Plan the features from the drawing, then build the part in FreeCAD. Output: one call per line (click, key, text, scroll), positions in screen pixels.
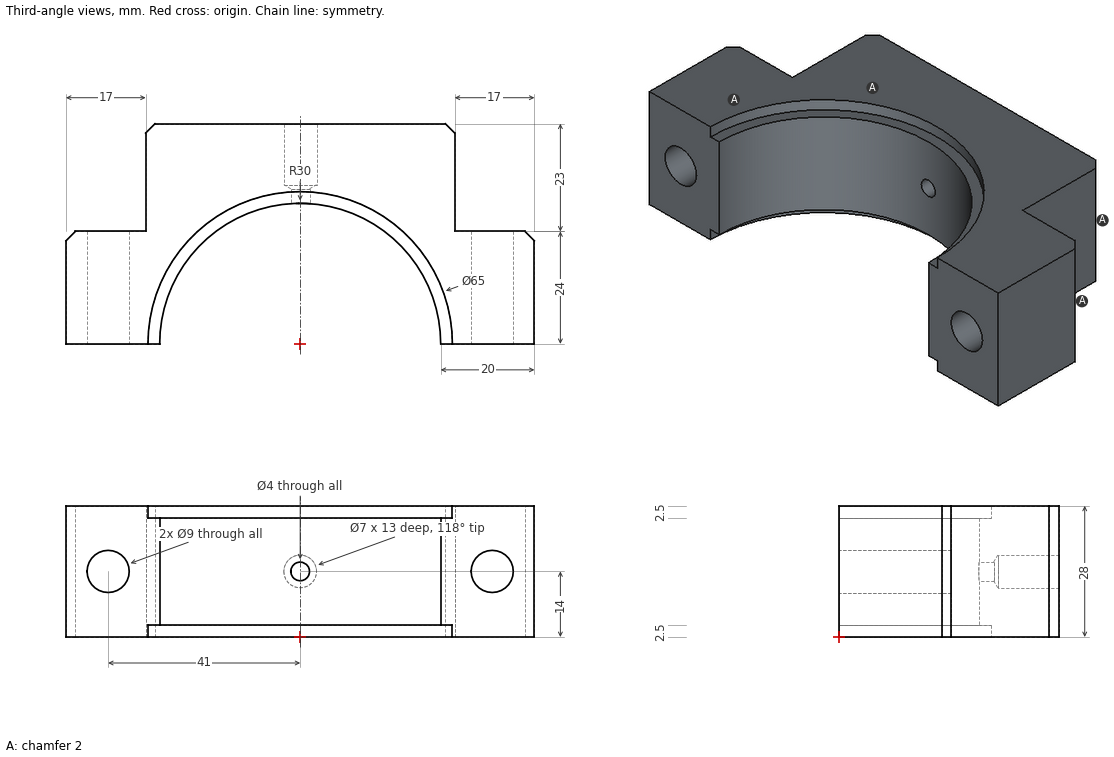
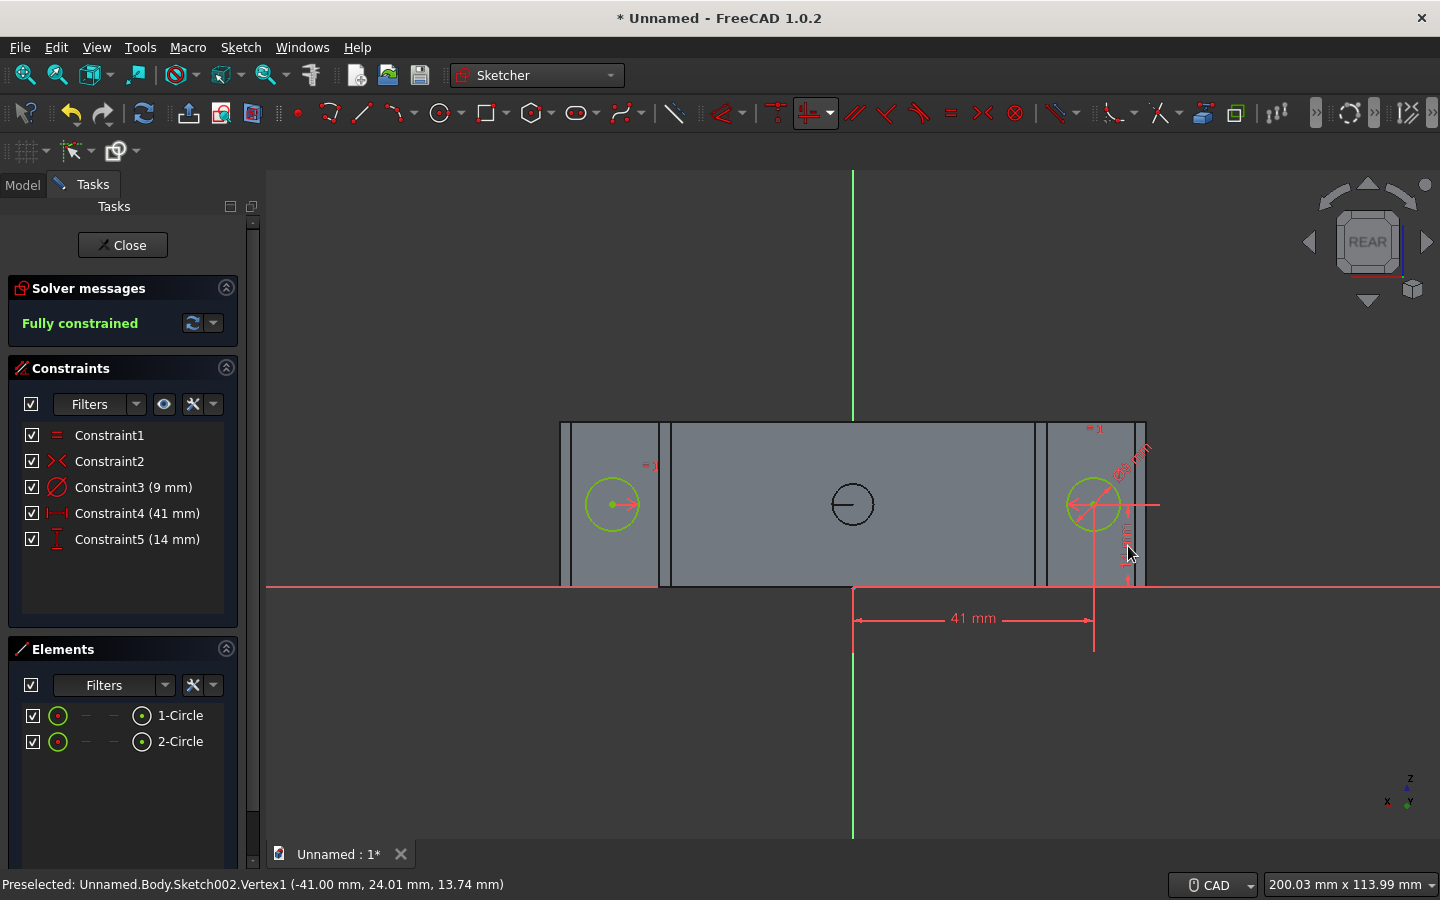
click(123, 245)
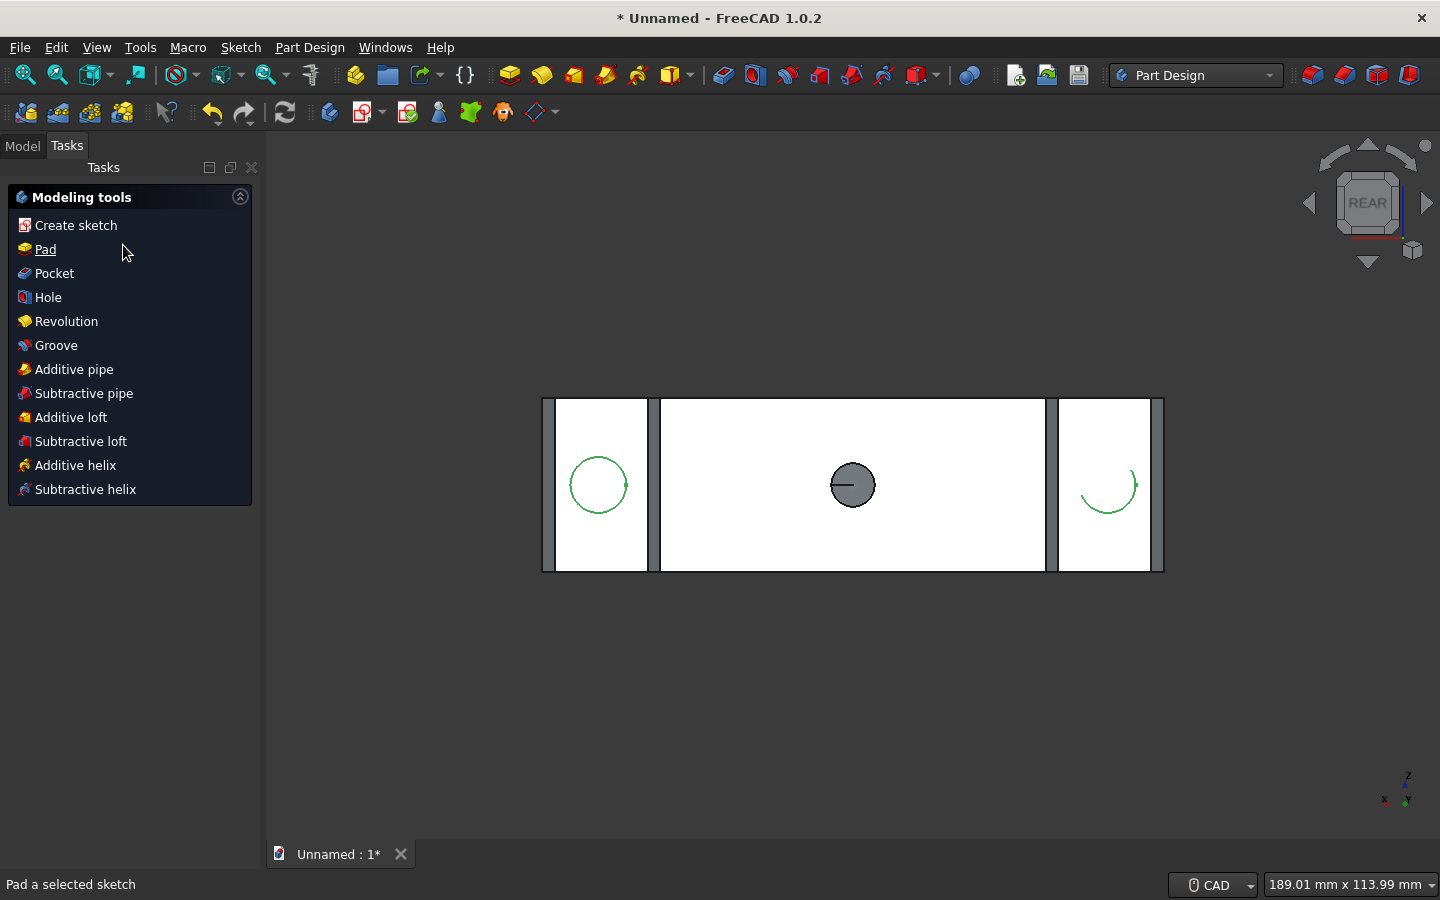
click(756, 76)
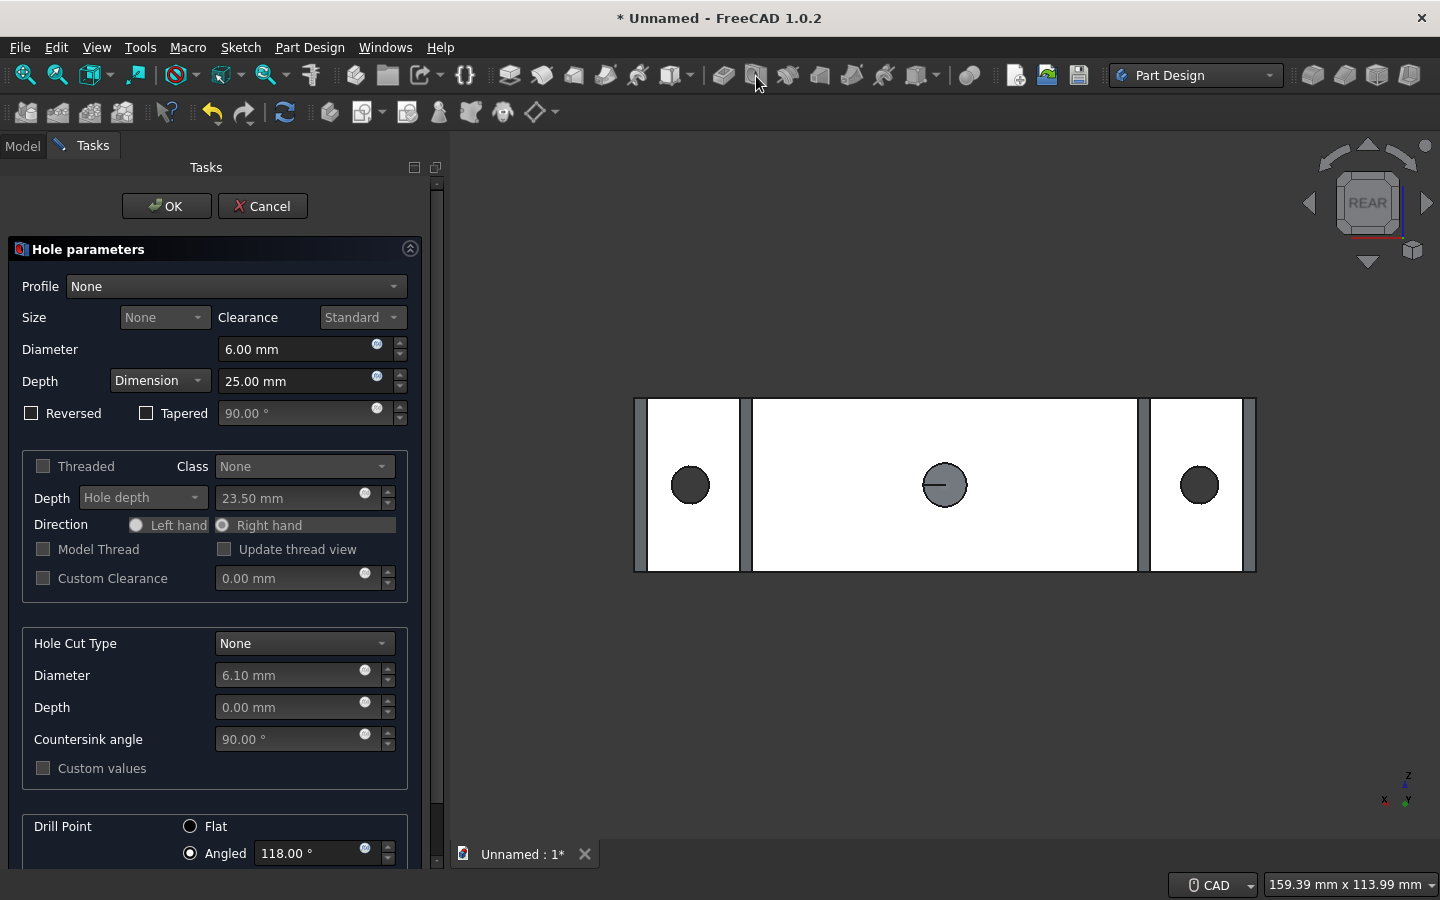
triple_click(305, 349)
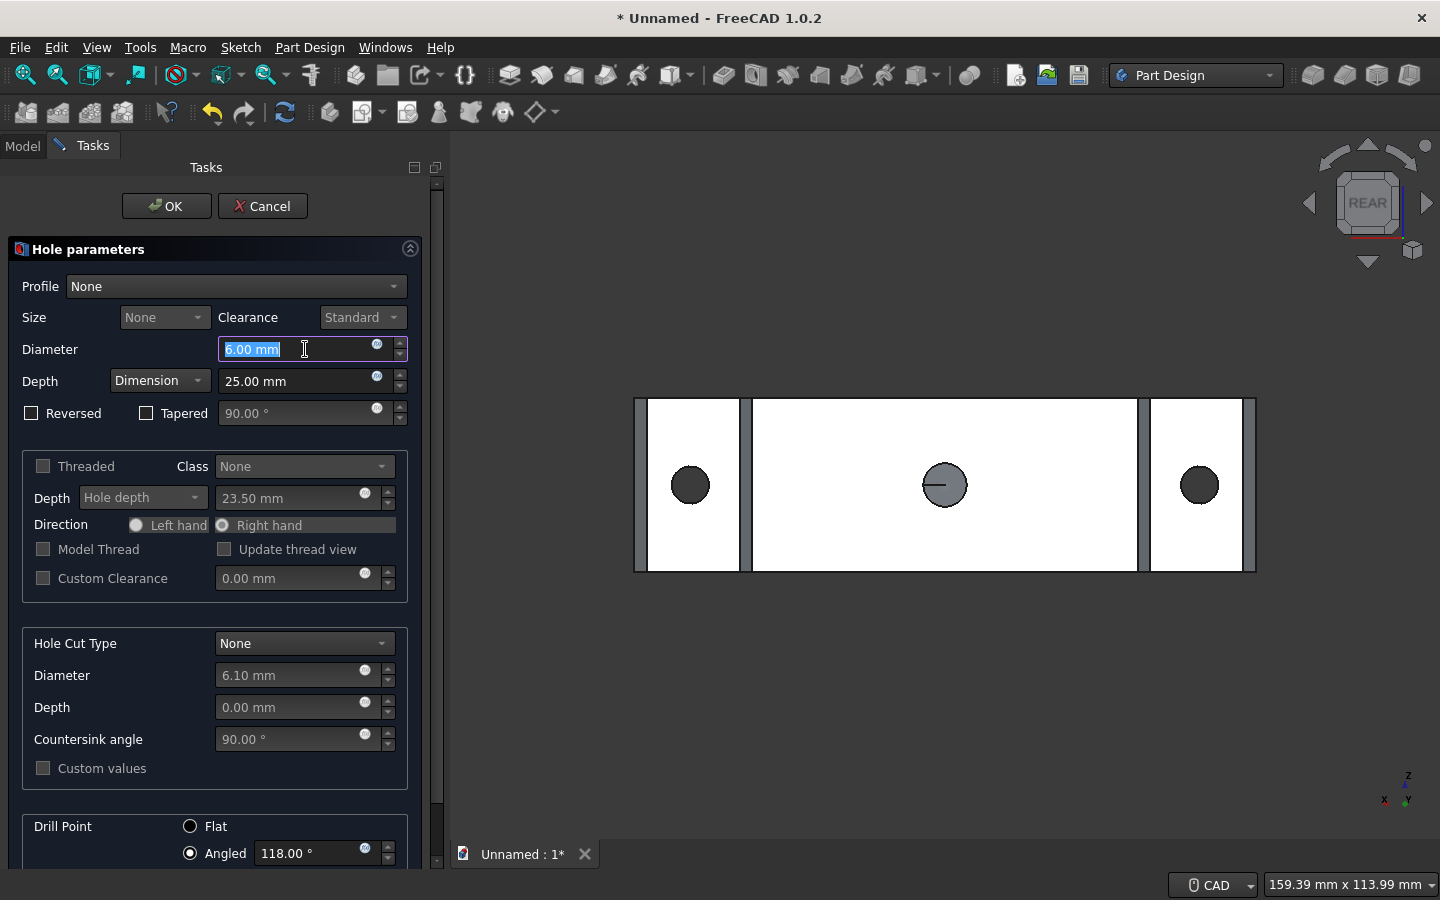
text(9)
key(Tab)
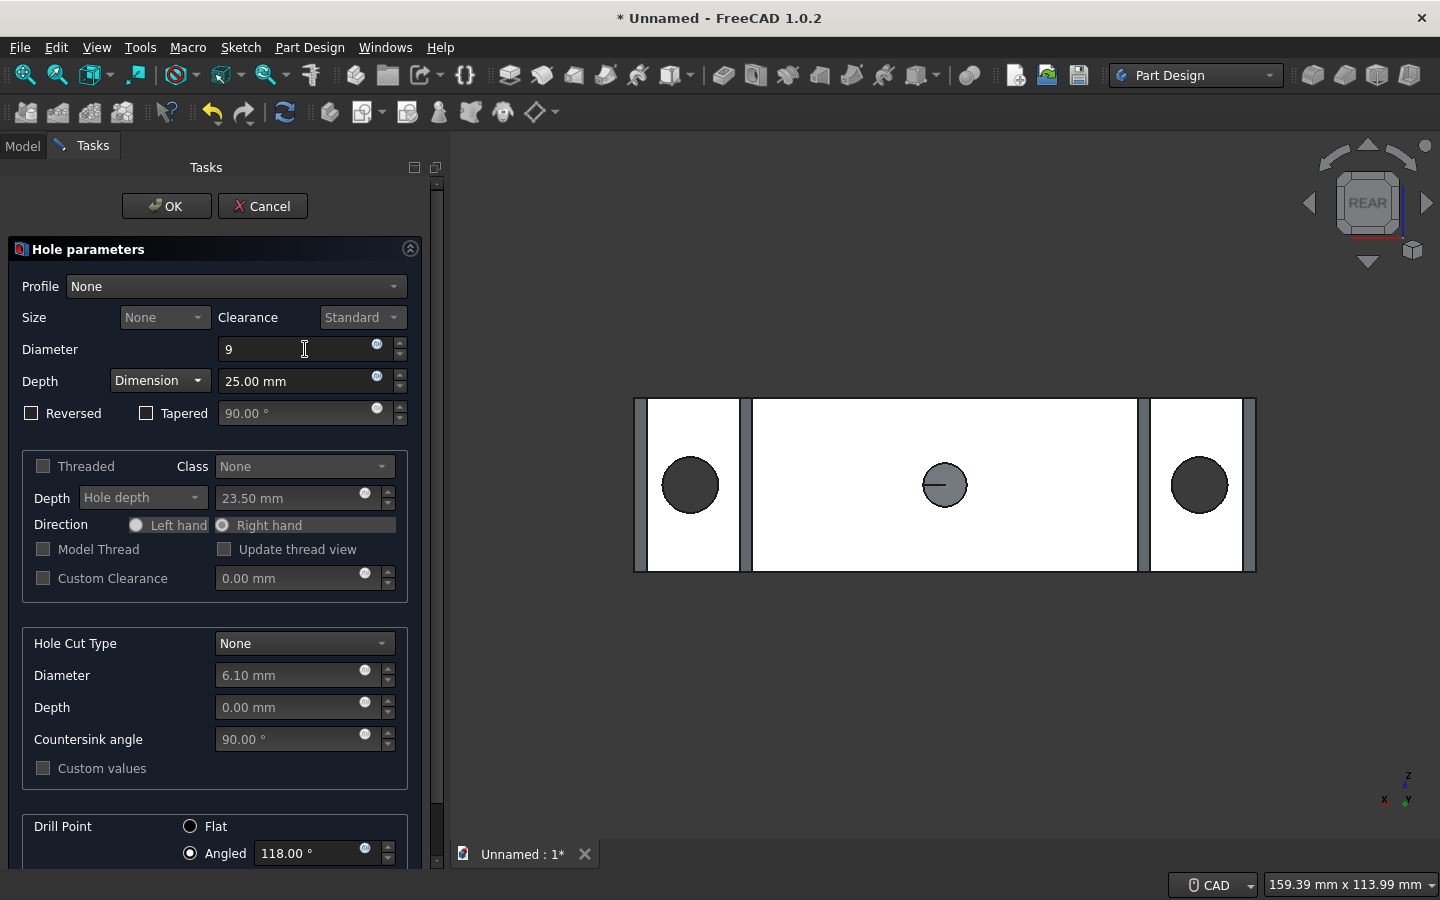
click(161, 380)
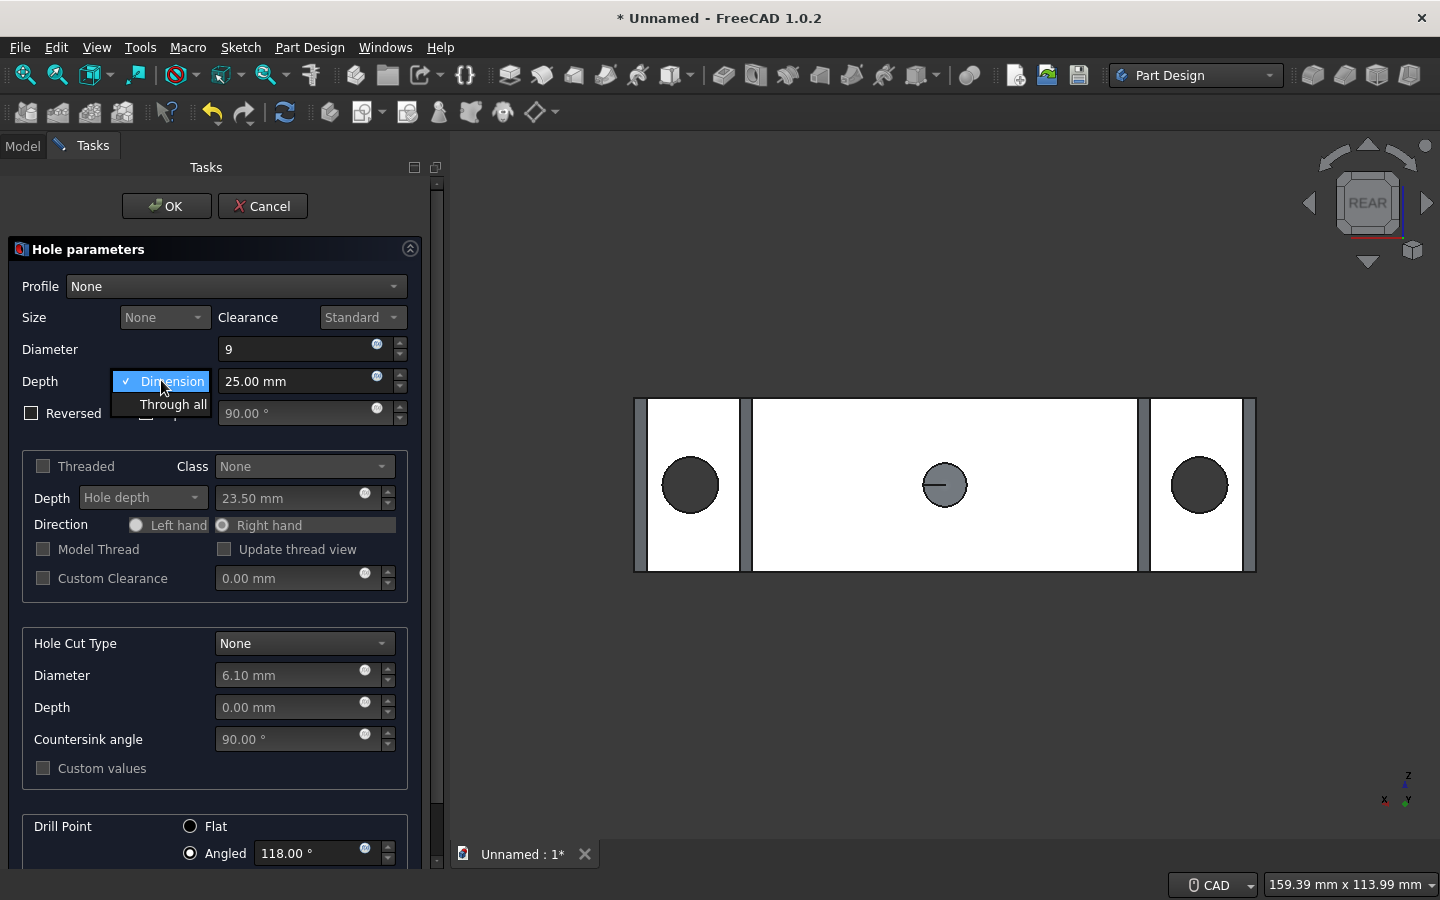
click(160, 404)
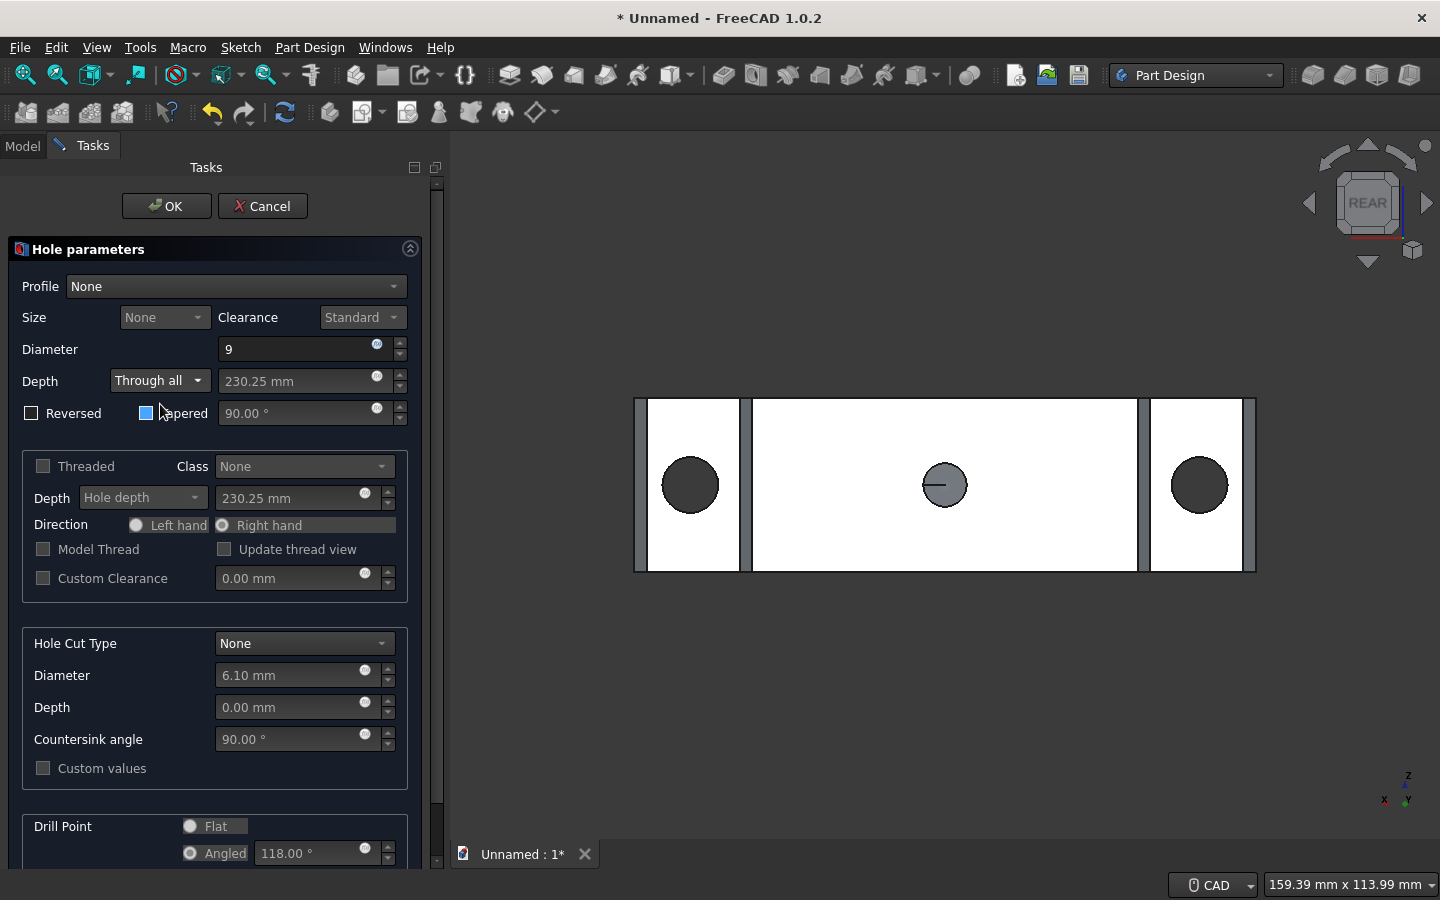
click(167, 206)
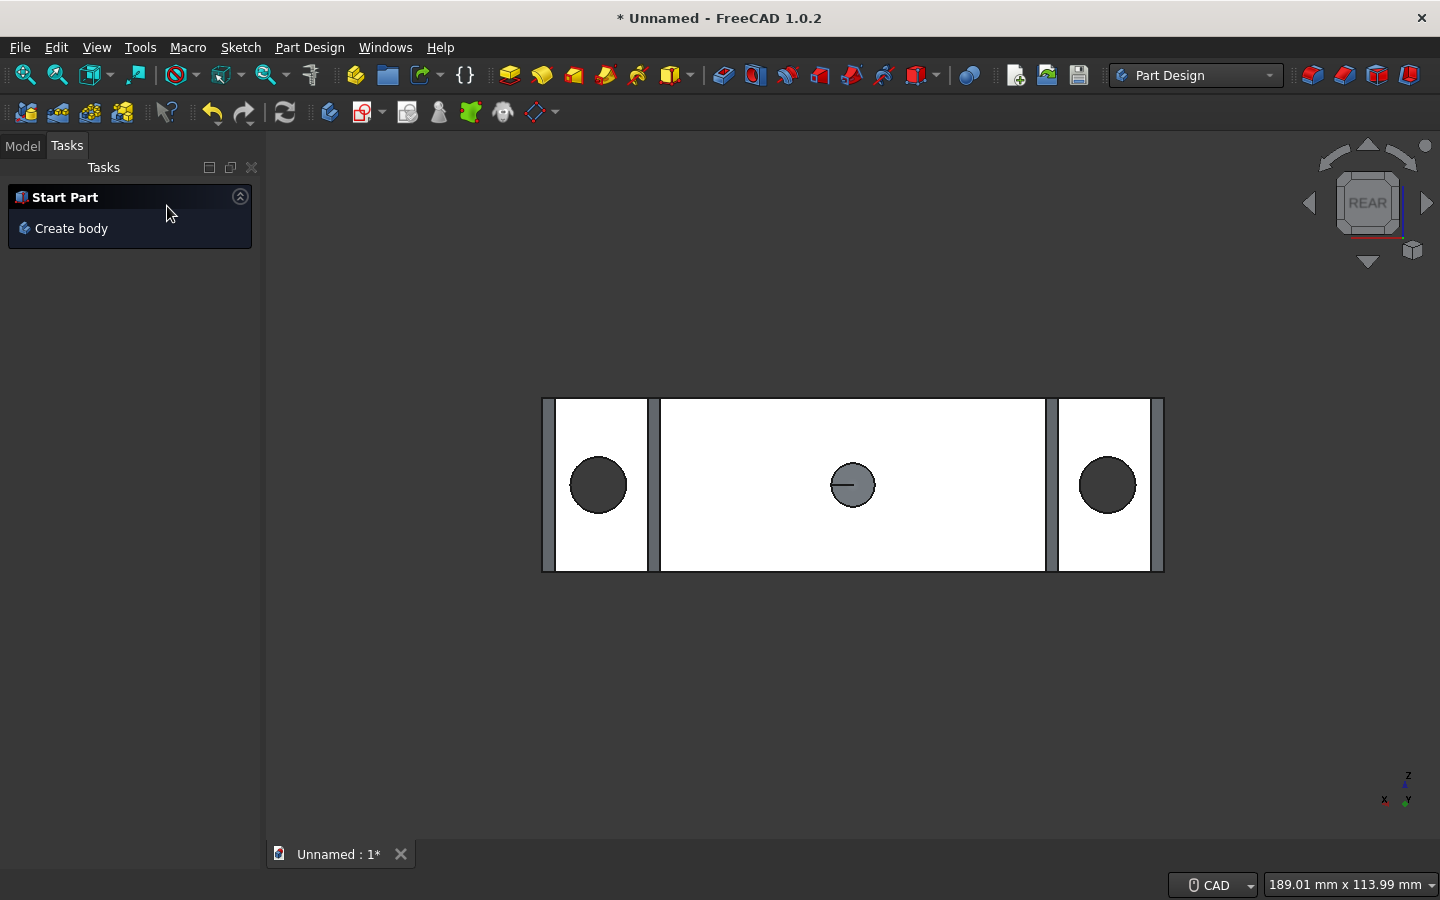
key(5)